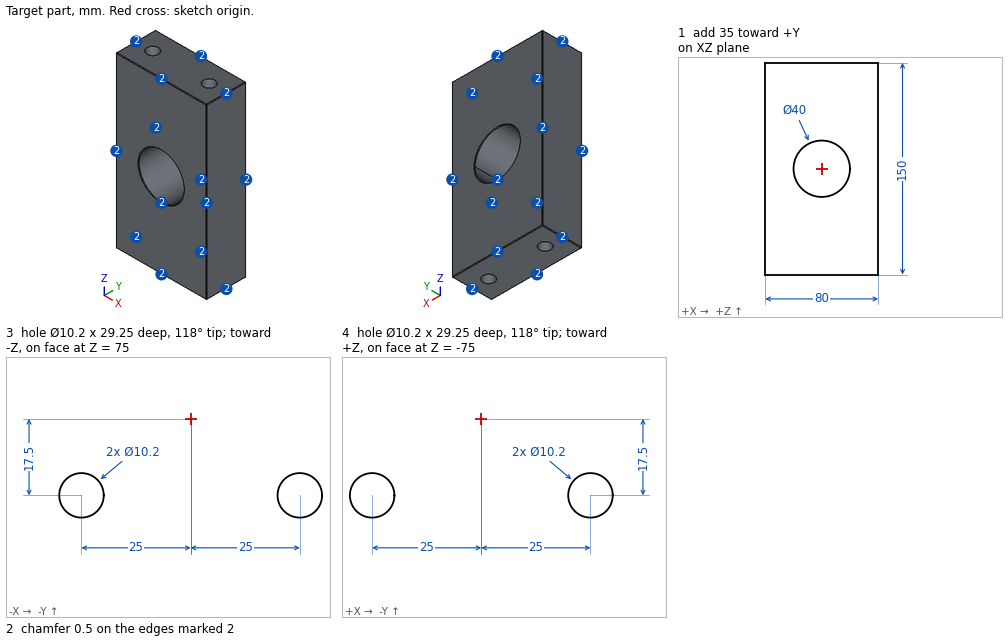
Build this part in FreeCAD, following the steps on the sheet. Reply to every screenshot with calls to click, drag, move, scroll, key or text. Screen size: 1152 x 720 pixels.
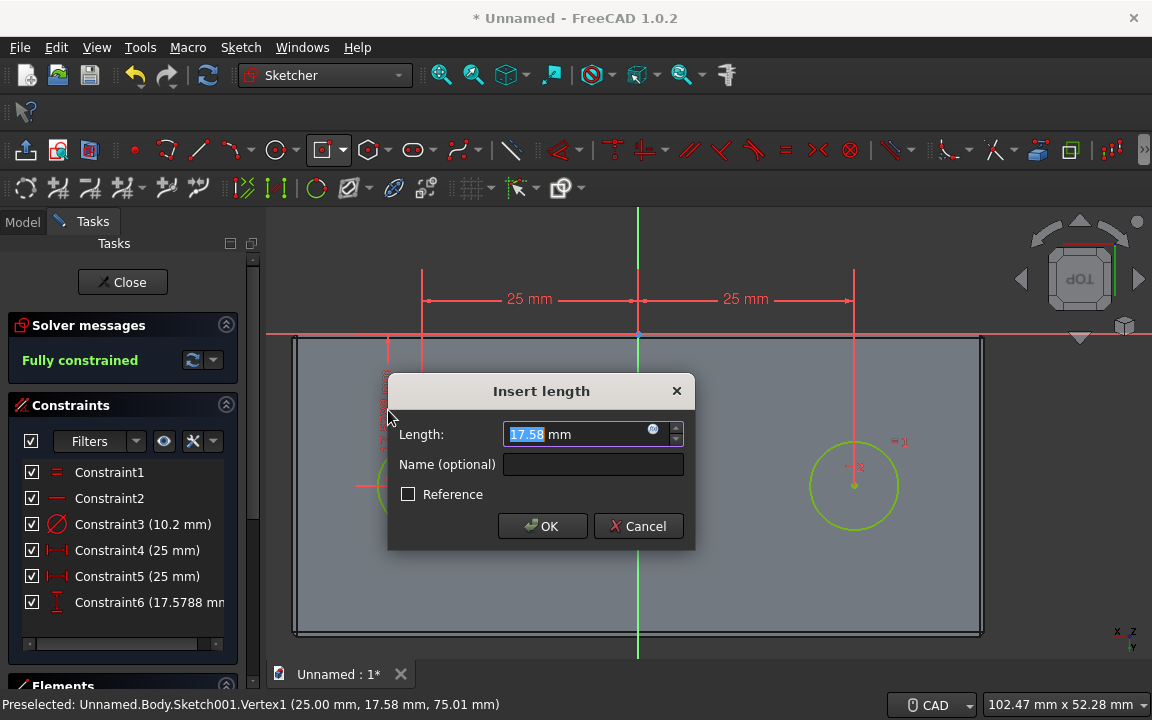
text(17.5)
key(Return)
key(Escape)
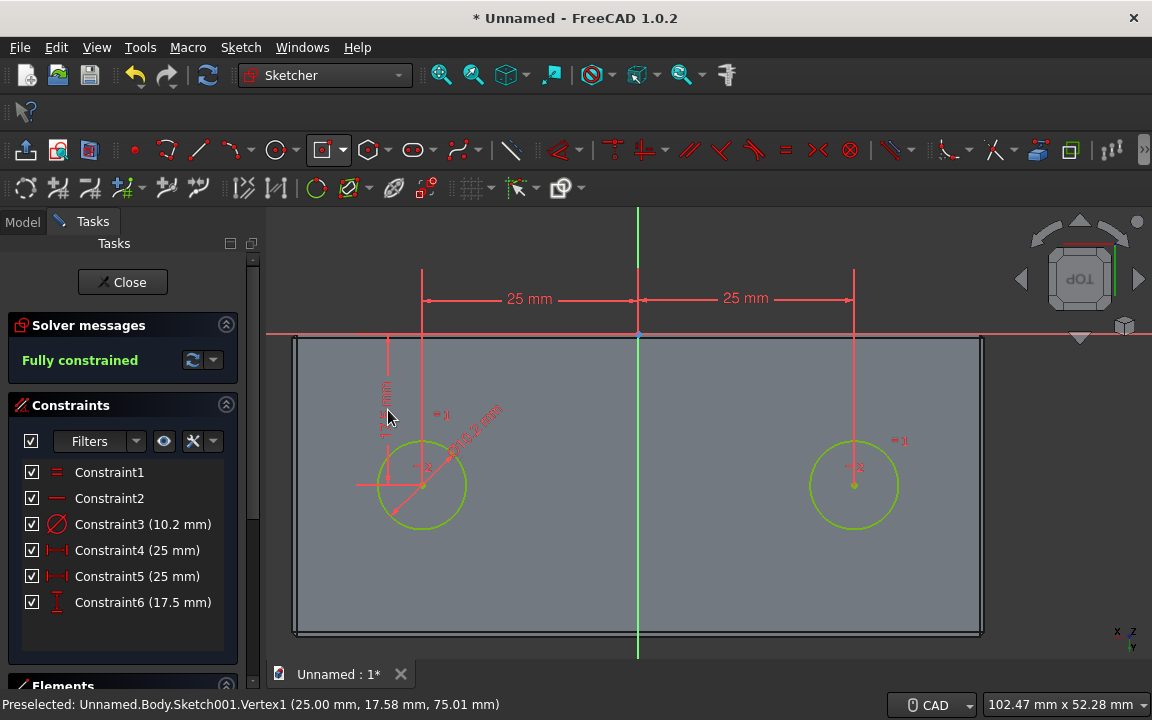
click(123, 282)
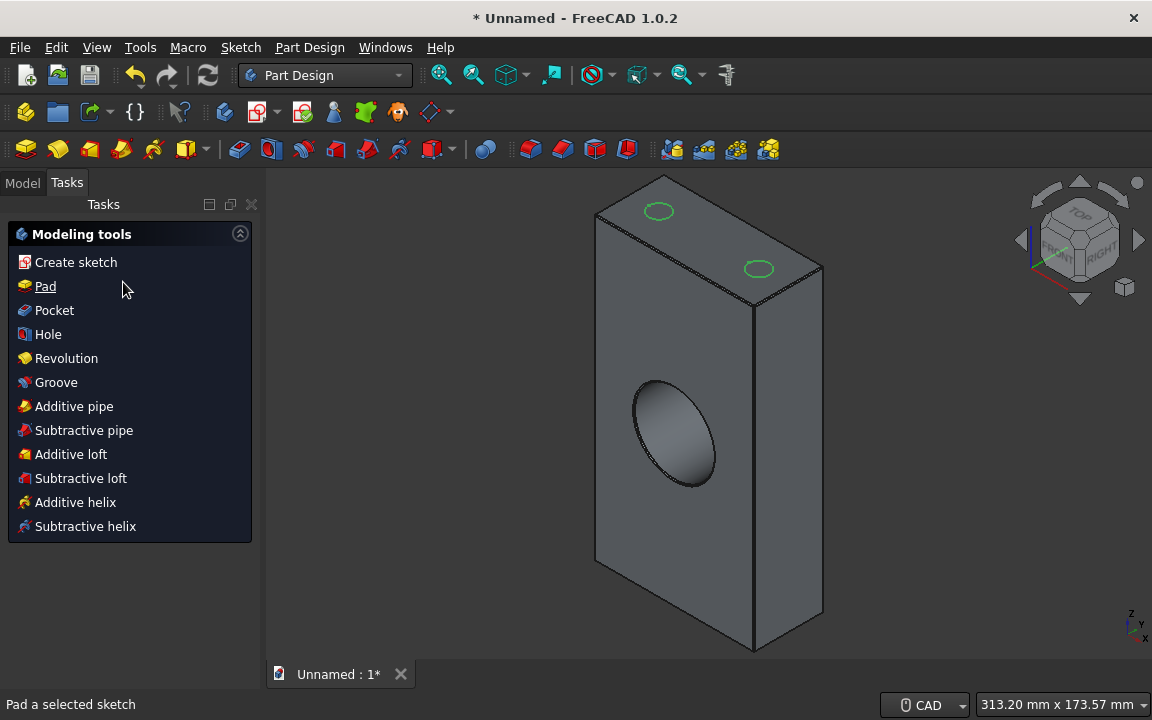
click(272, 150)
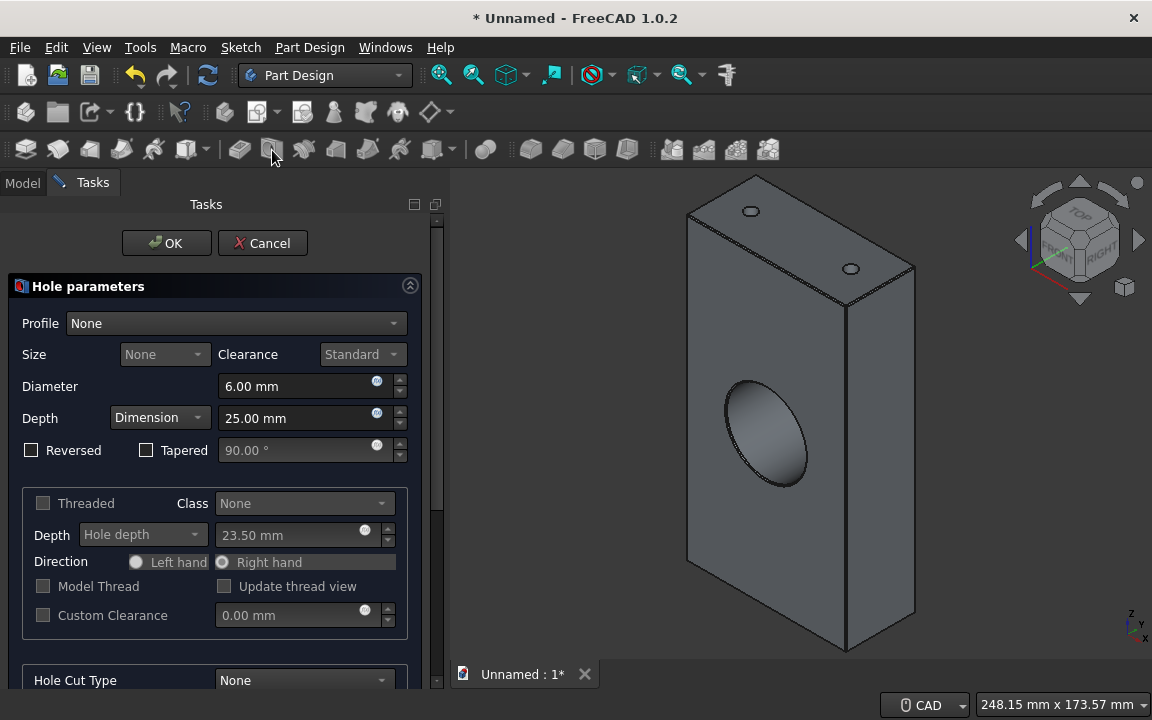
triple_click(305, 386)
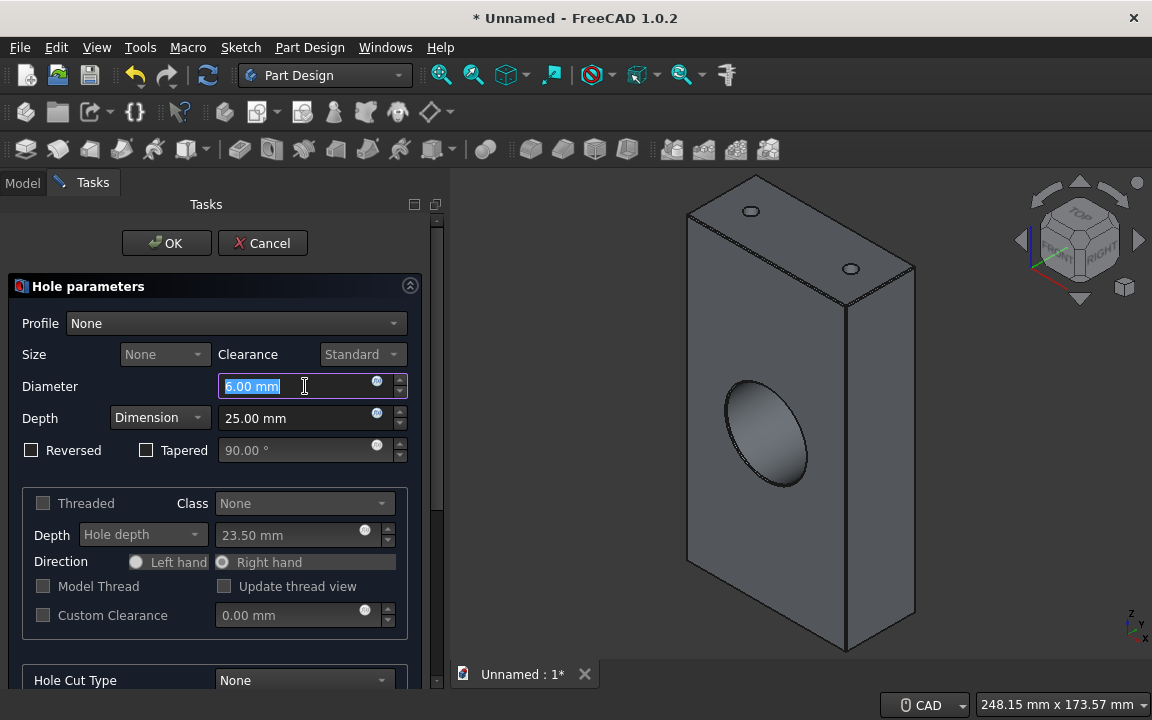
text(10.2)
key(Tab)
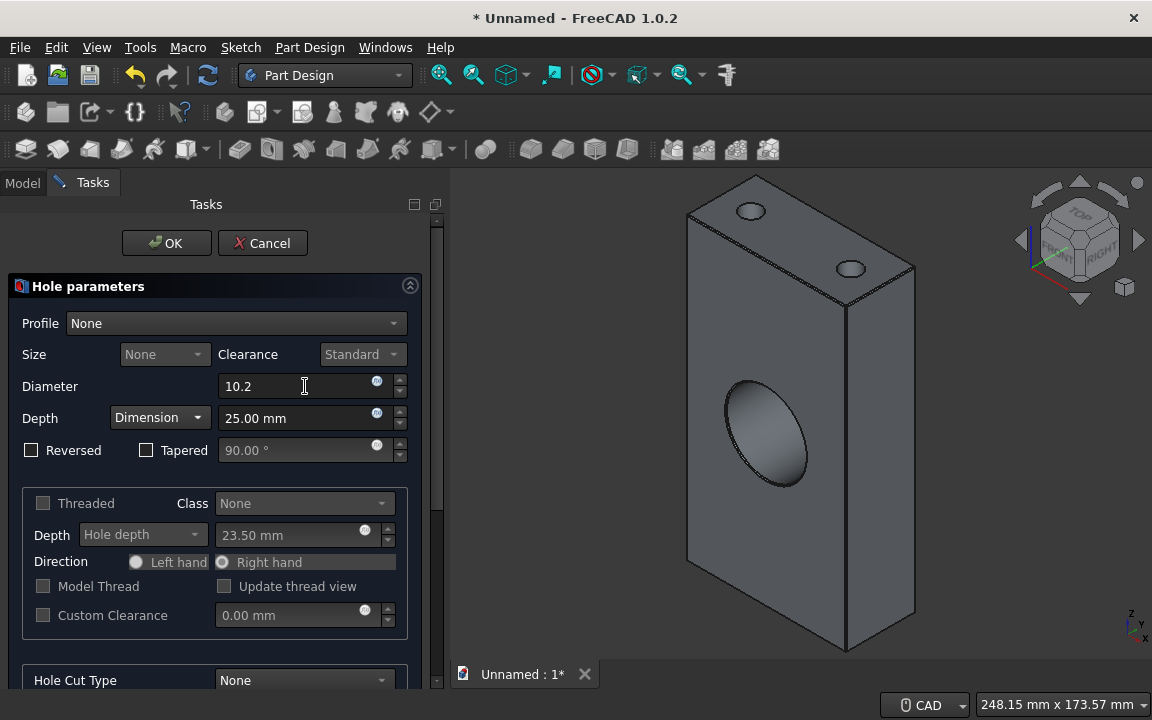
triple_click(305, 418)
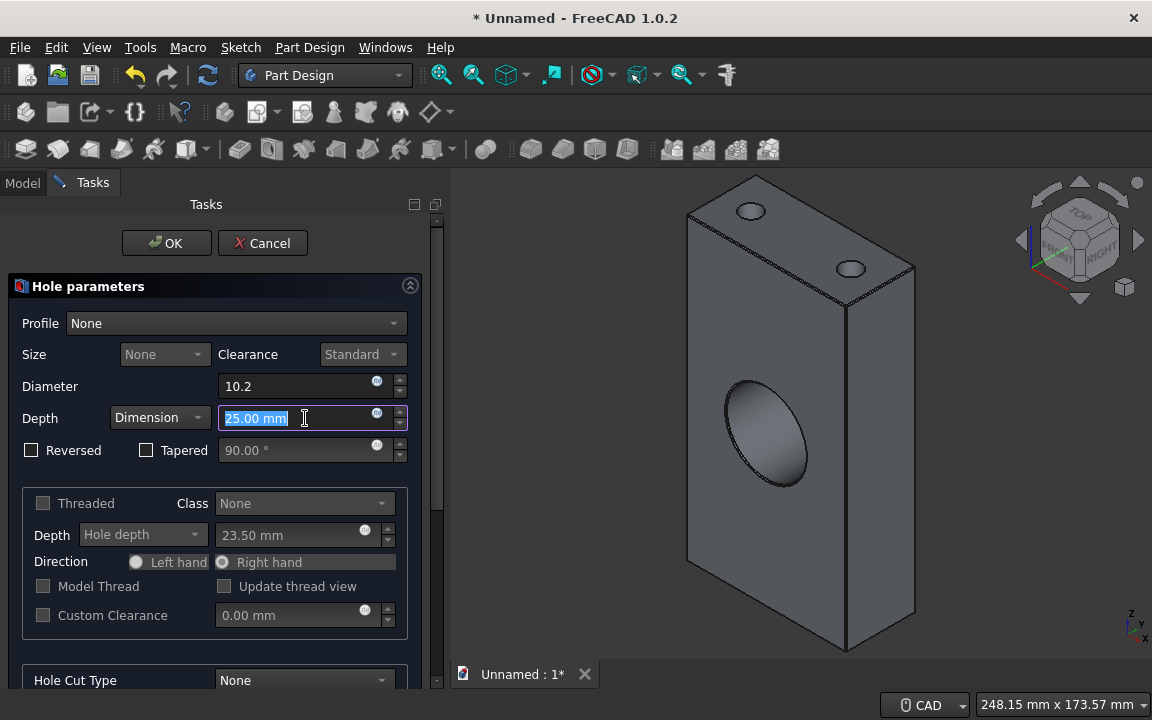
text(29.25)
key(Tab)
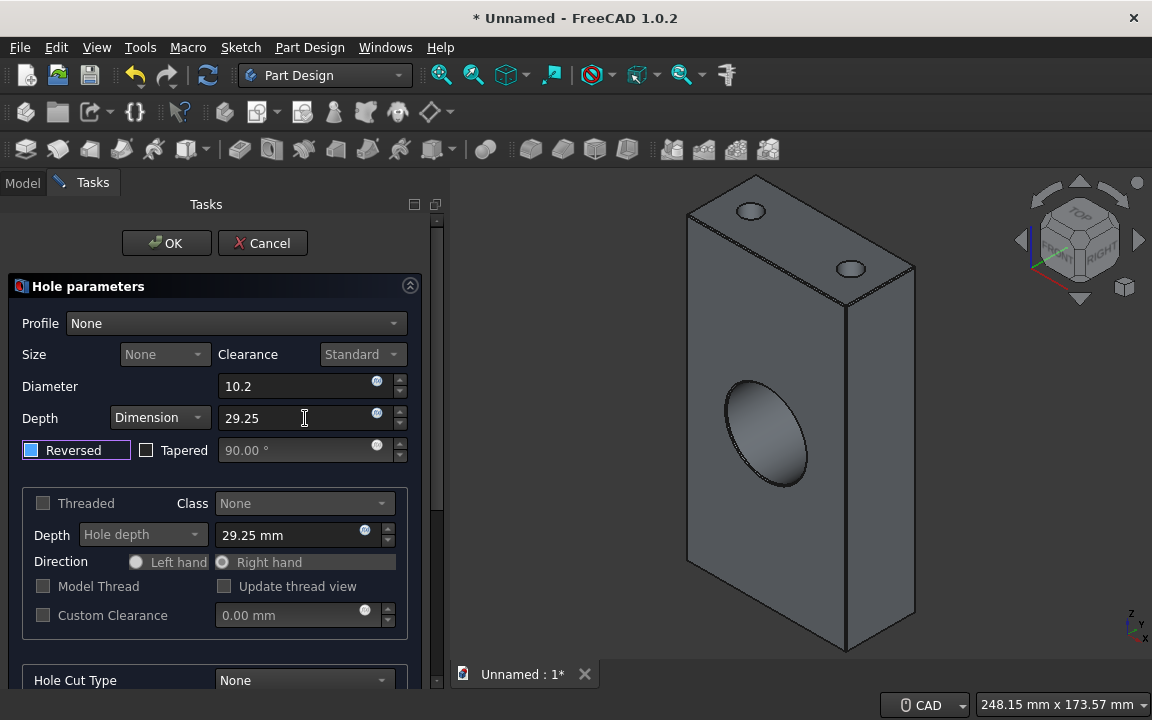
click(167, 243)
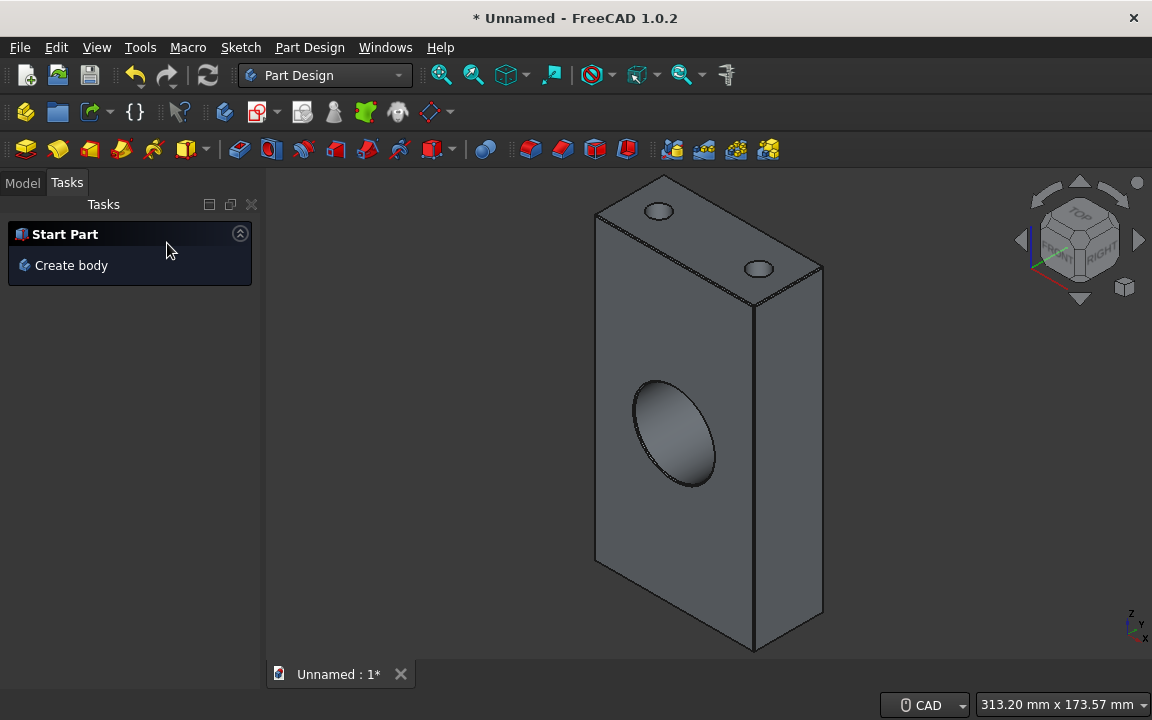
key(5)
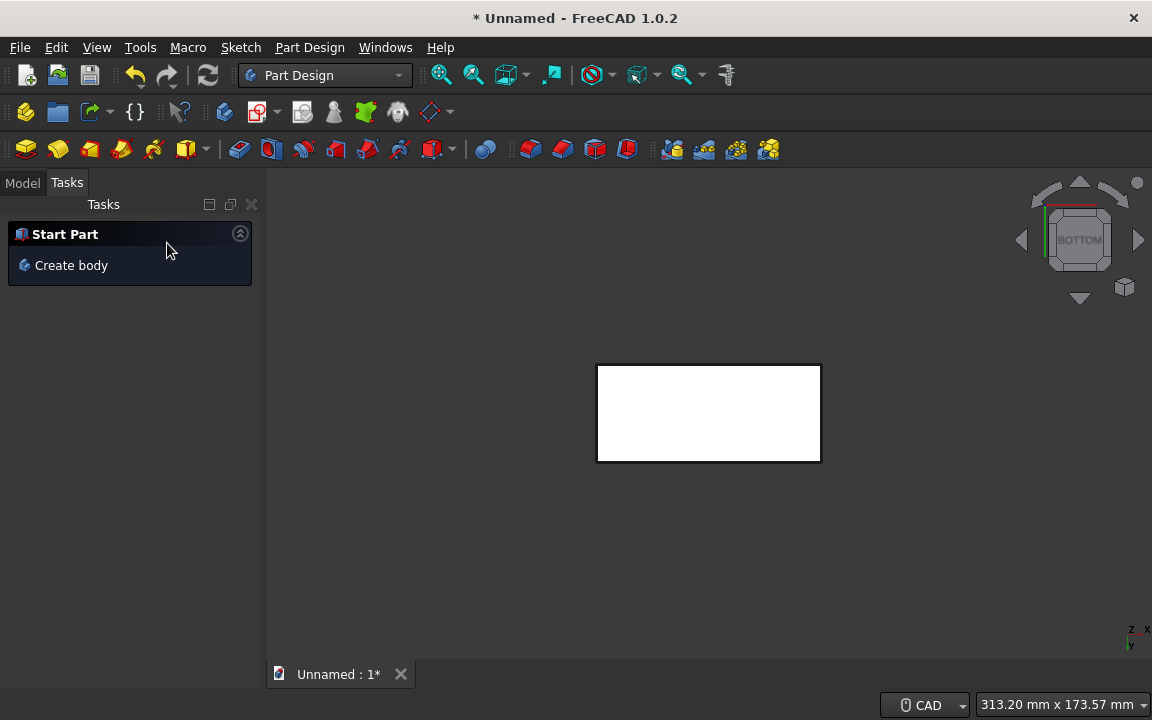
click(442, 76)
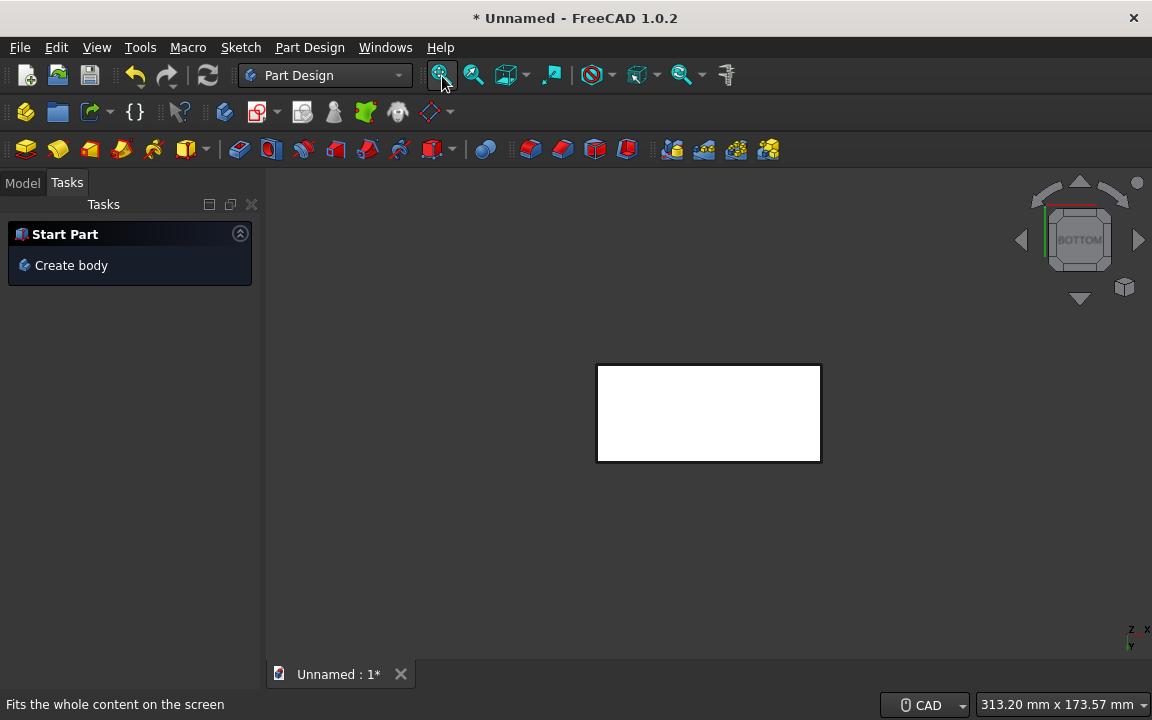
click(741, 412)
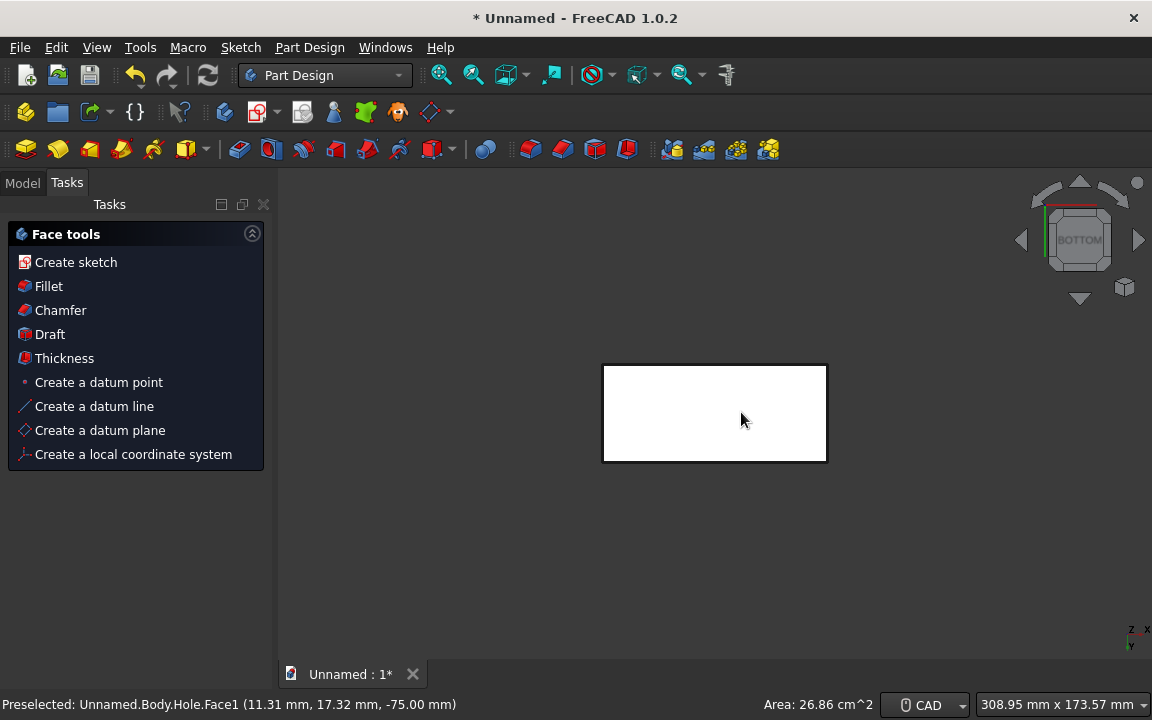
click(258, 112)